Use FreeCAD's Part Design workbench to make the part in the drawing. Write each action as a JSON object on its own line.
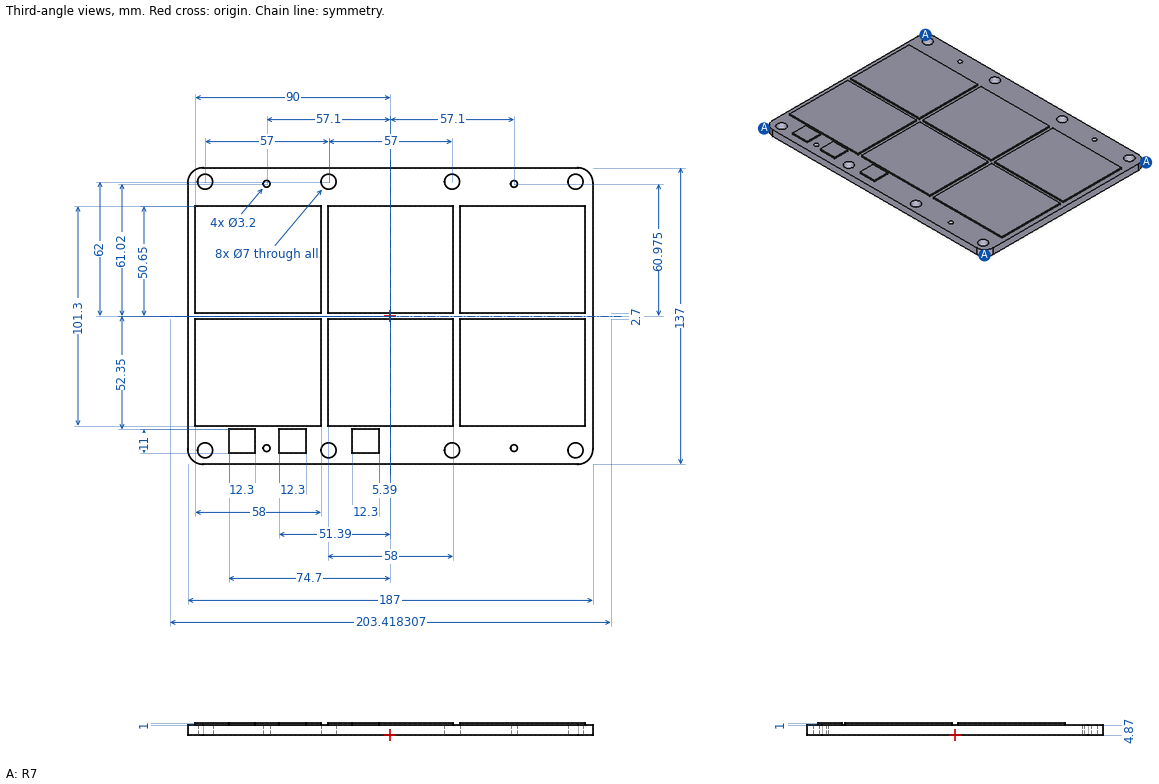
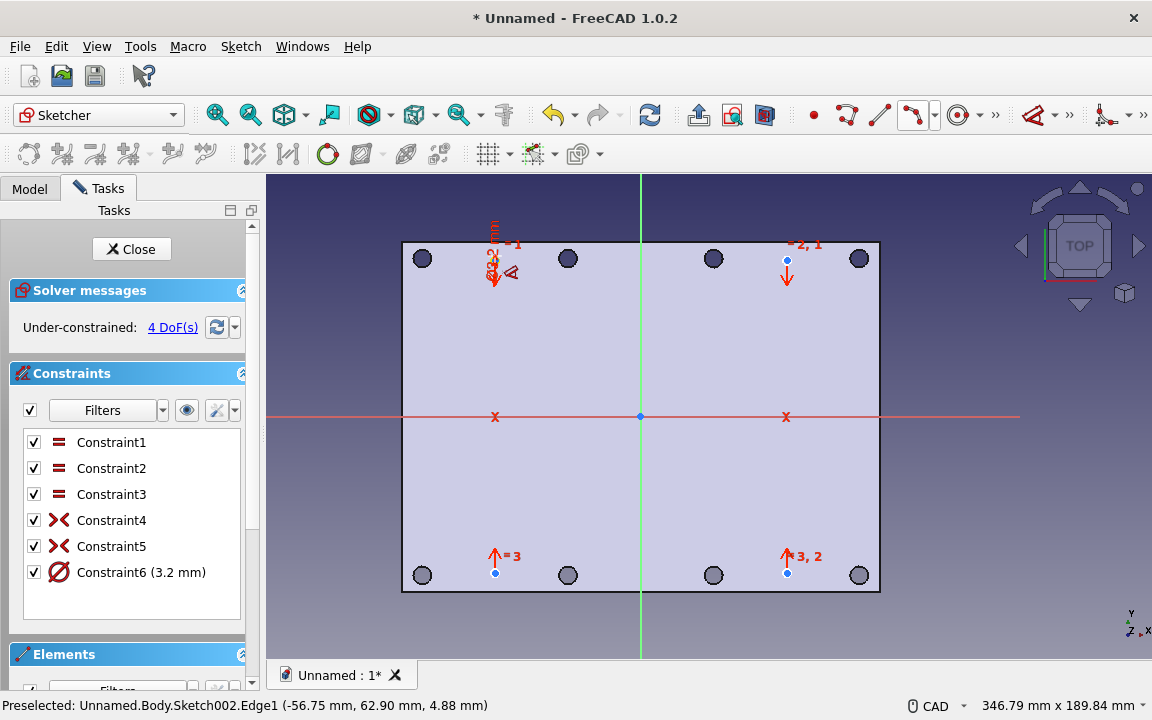
{"action": "left_click", "coordinate": [495, 261]}
{"action": "left_click", "coordinate": [568, 227]}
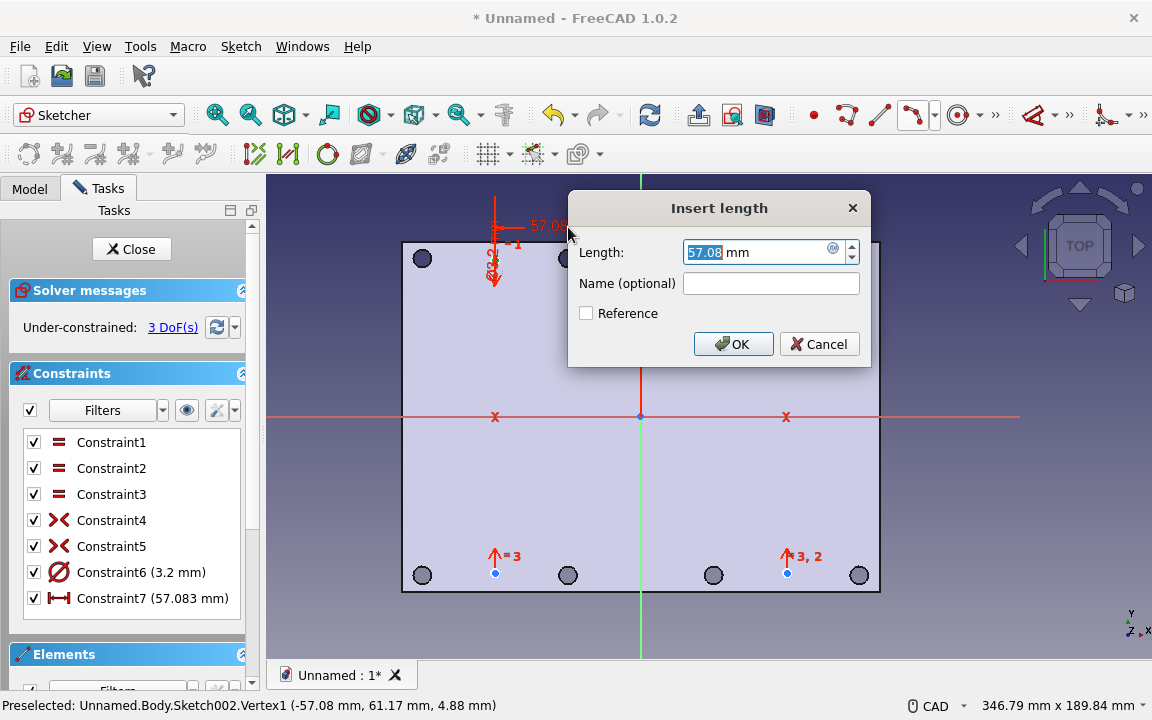
{"action": "type", "text": "57.1"}
{"action": "key", "text": "Return"}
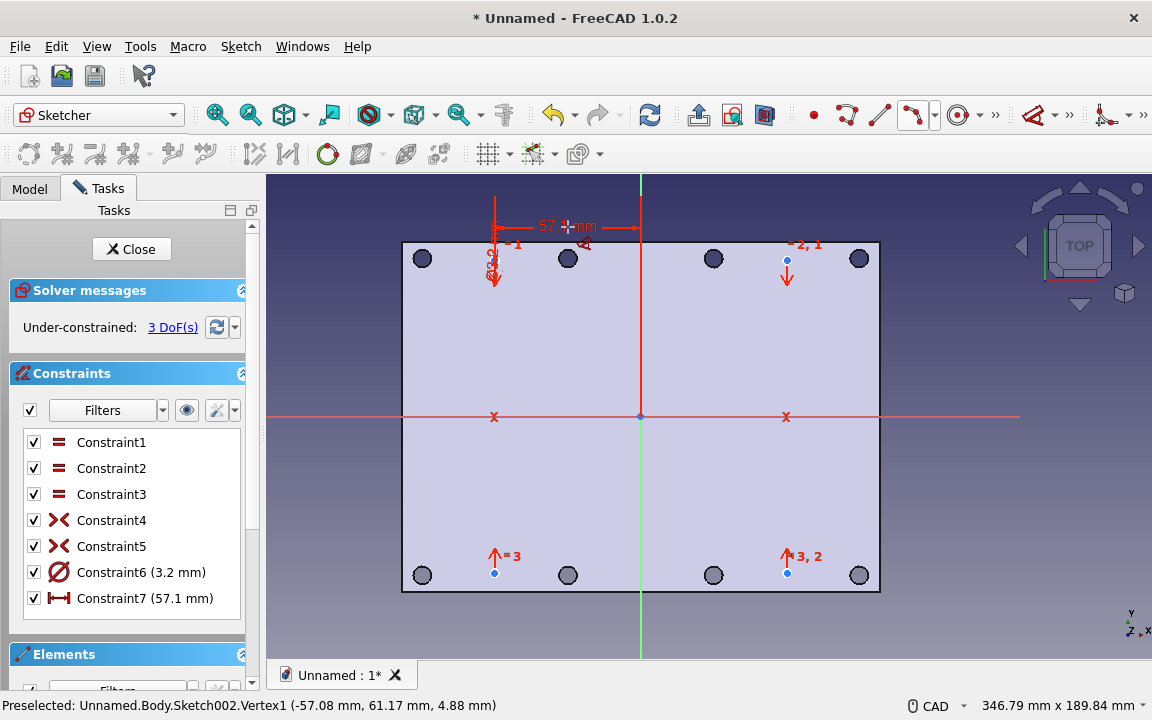
{"action": "left_click", "coordinate": [787, 261]}
{"action": "left_click", "coordinate": [714, 227]}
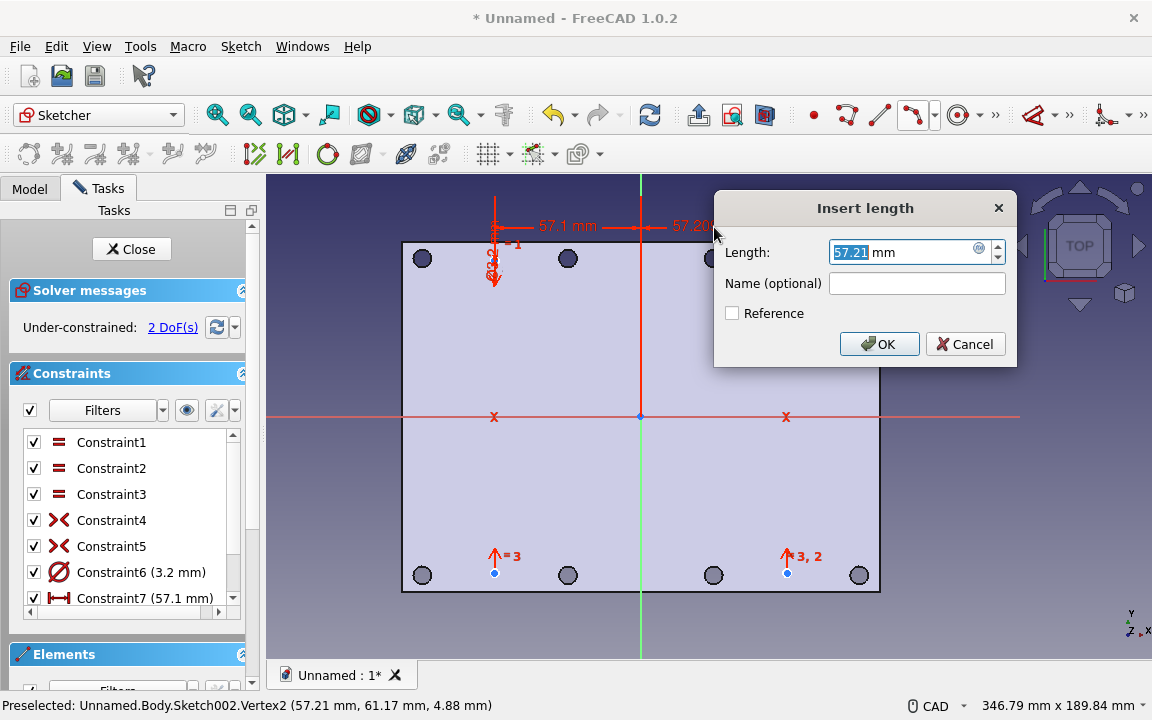
{"action": "type", "text": "57.1"}
{"action": "key", "text": "Return"}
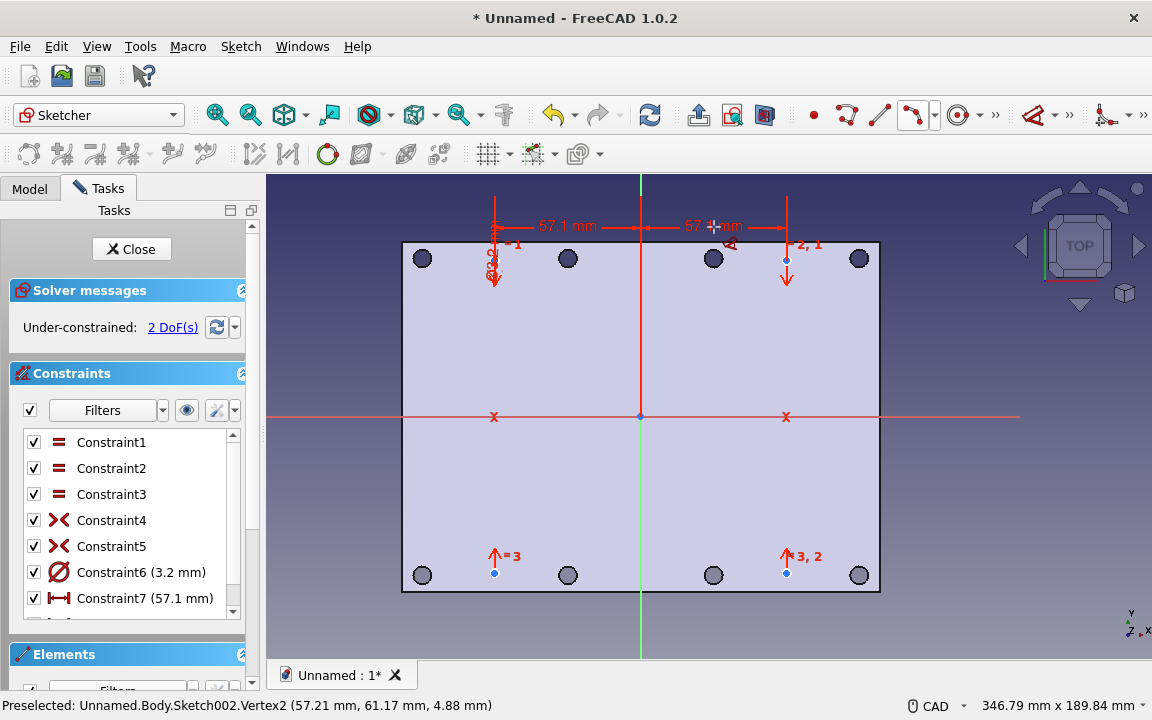
{"action": "left_click", "coordinate": [495, 261]}
{"action": "left_click", "coordinate": [461, 339]}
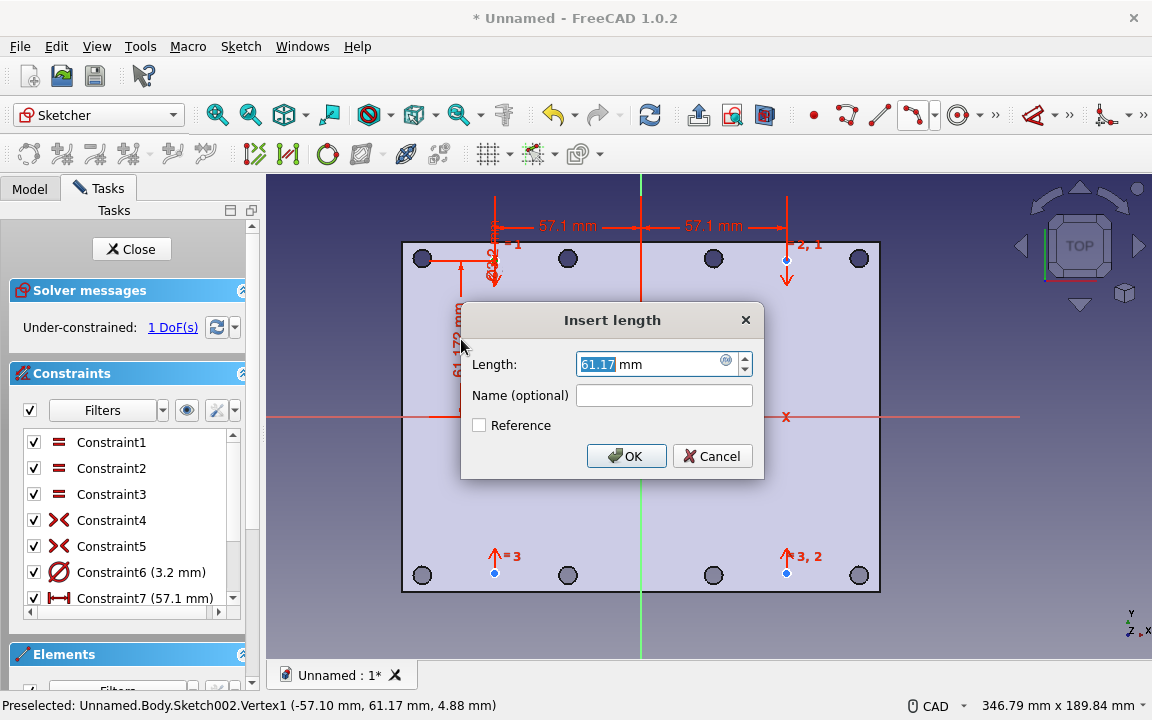
{"action": "type", "text": "61.02"}
{"action": "key", "text": "Return"}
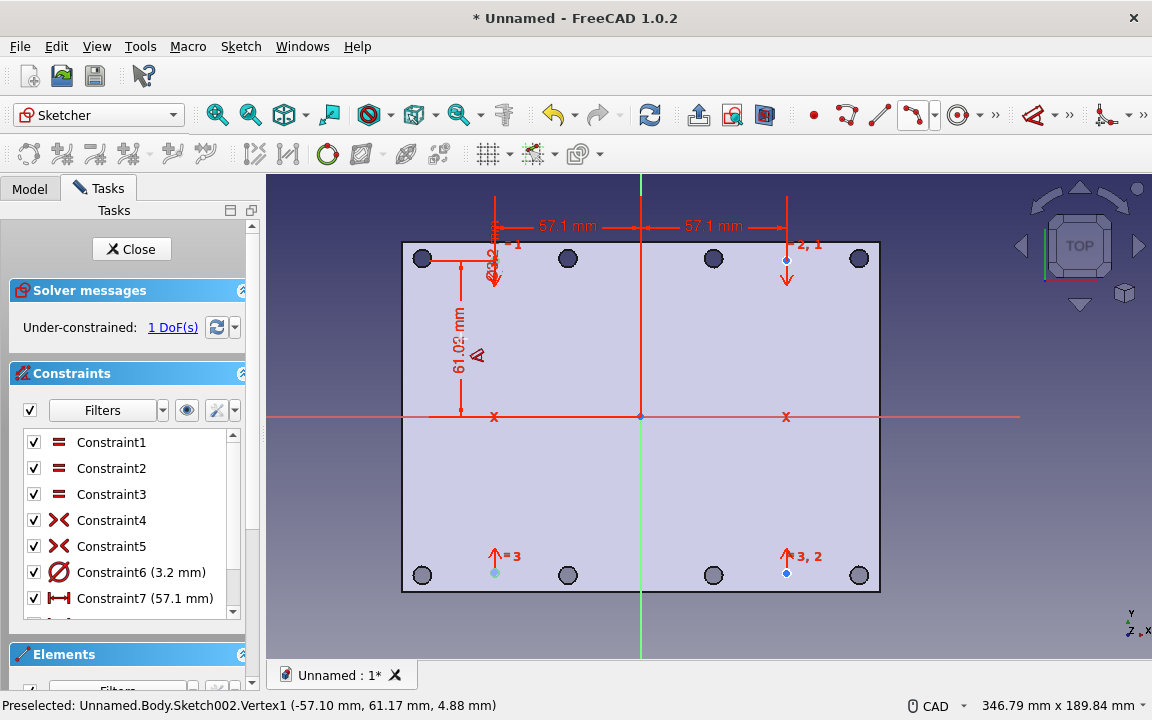
{"action": "left_click", "coordinate": [787, 261]}
{"action": "left_click", "coordinate": [821, 339]}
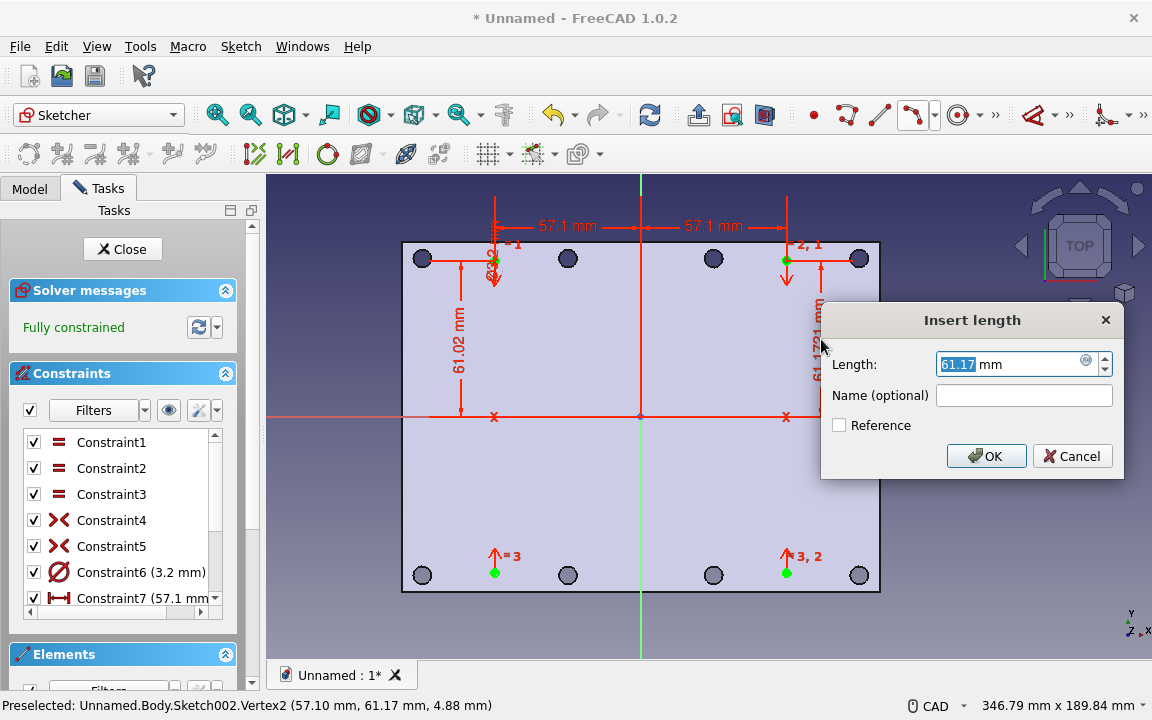
{"action": "type", "text": "60.975"}
{"action": "key", "text": "Return"}
{"action": "key", "text": "Escape"}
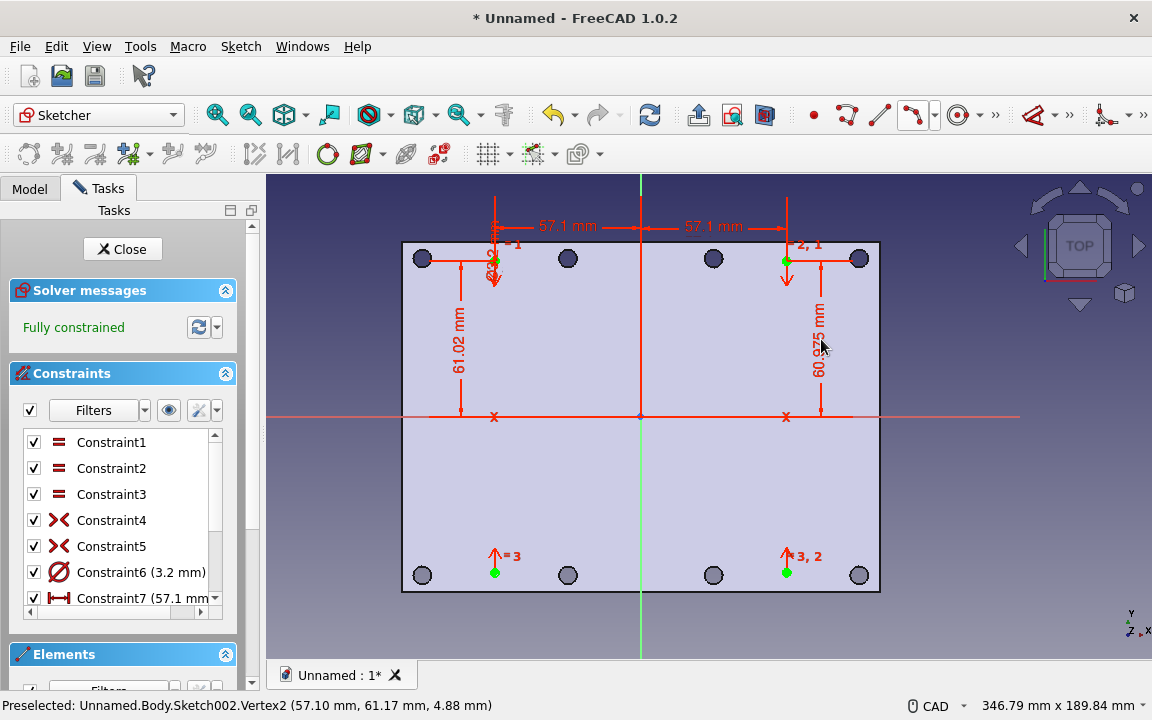
{"action": "left_click", "coordinate": [123, 249]}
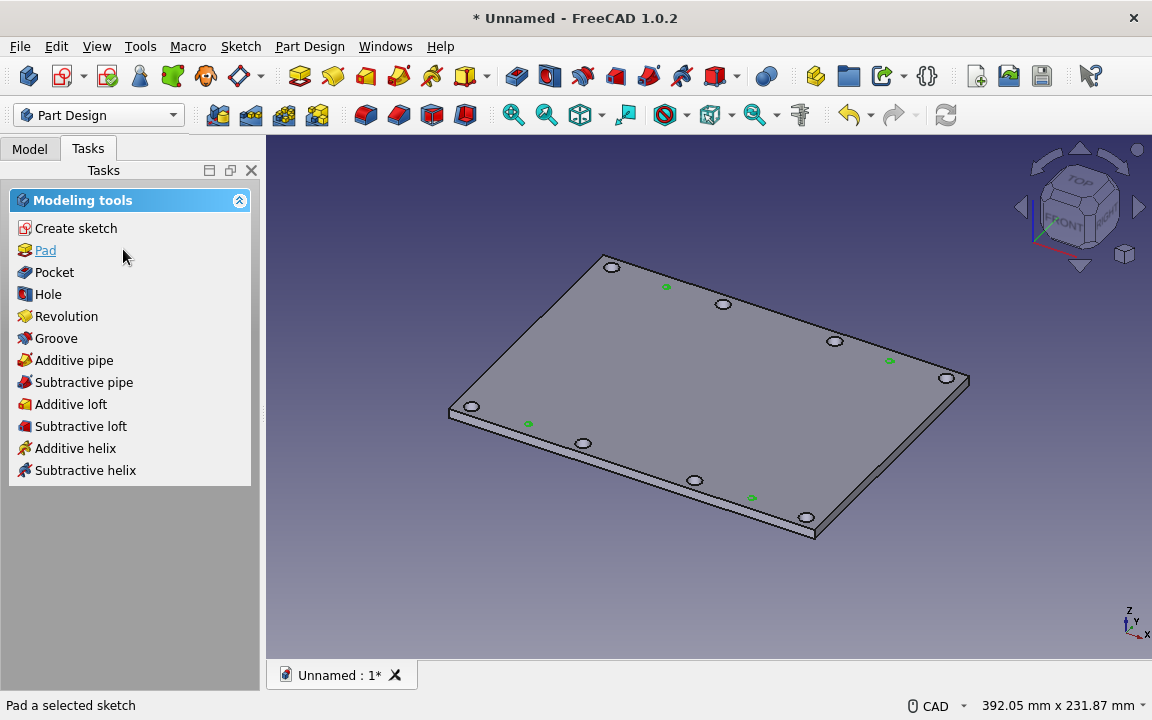
{"action": "left_click", "coordinate": [517, 76]}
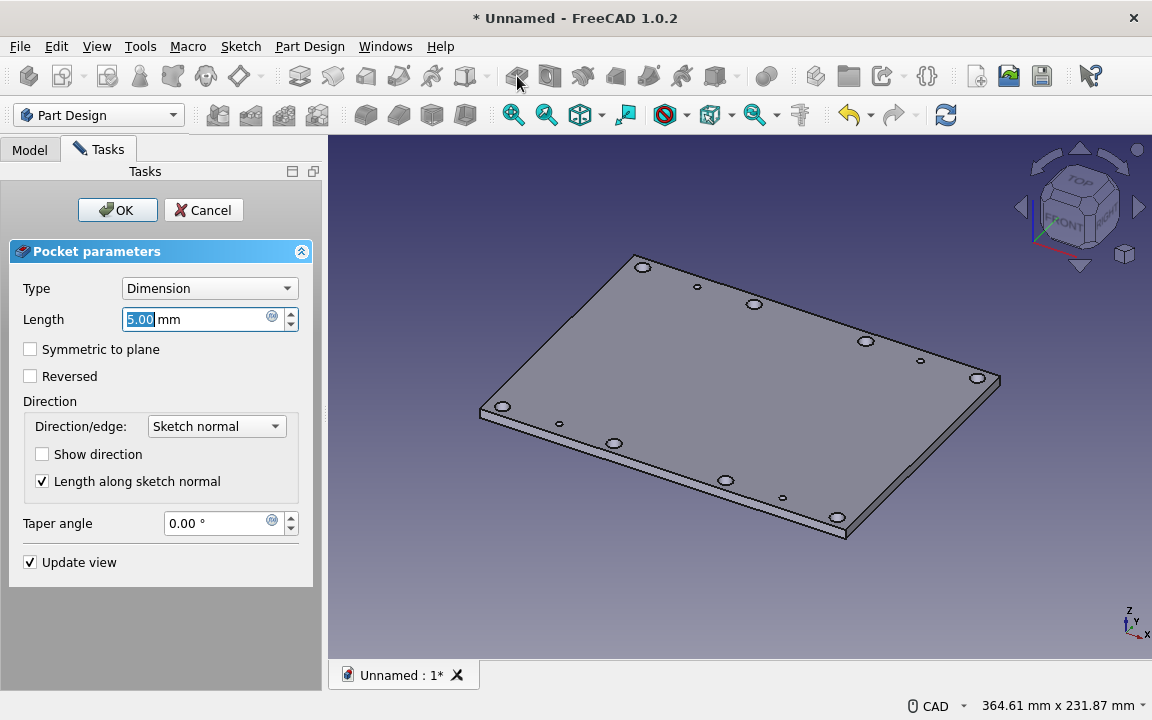
{"action": "left_click", "coordinate": [210, 288]}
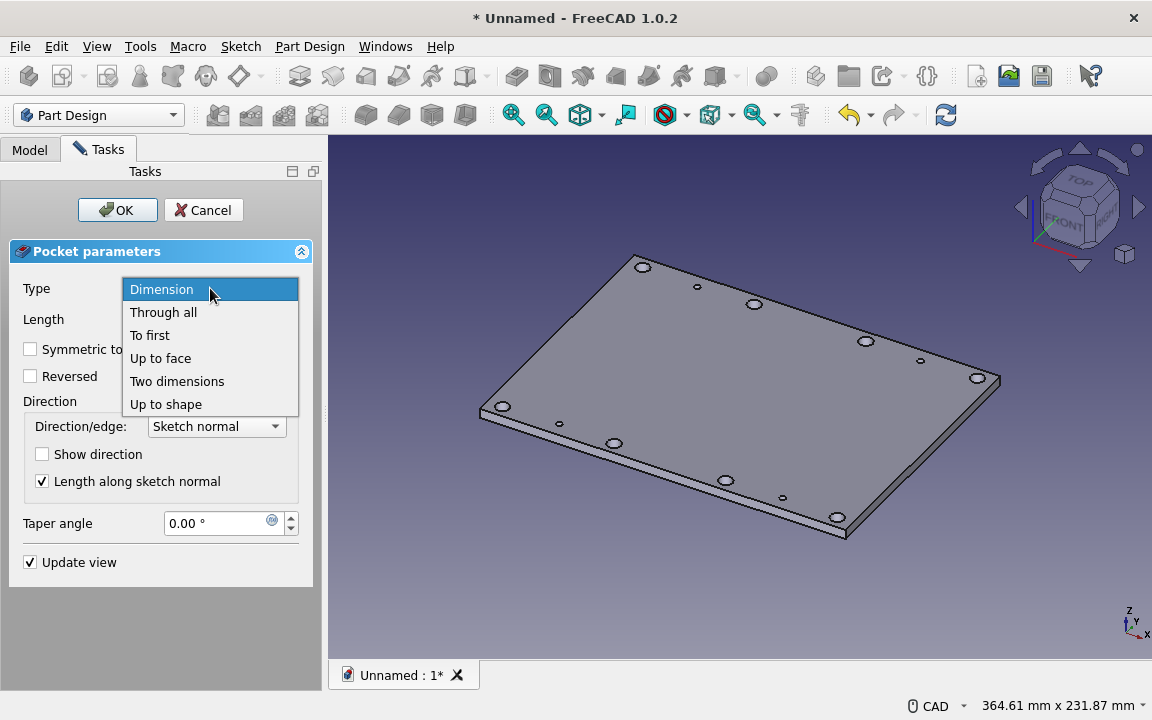
{"action": "left_click", "coordinate": [208, 312]}